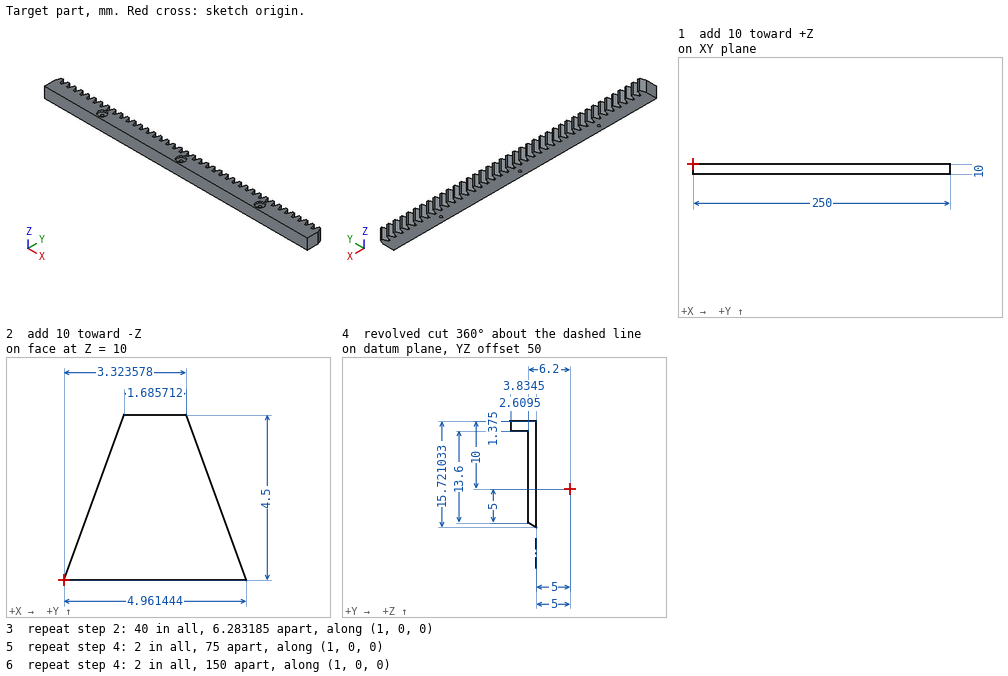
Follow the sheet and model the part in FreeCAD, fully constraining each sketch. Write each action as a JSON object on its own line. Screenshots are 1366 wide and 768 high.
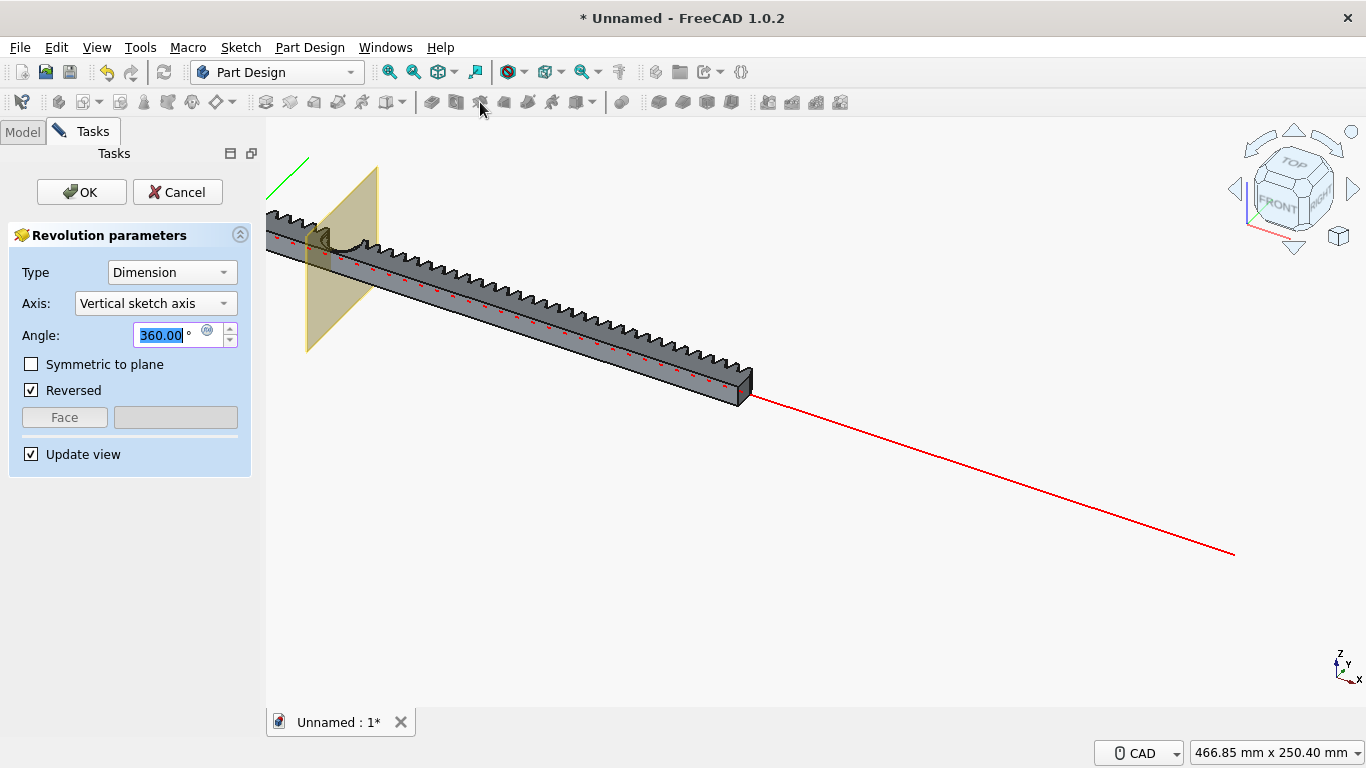
{"action": "left_click", "coordinate": [156, 304]}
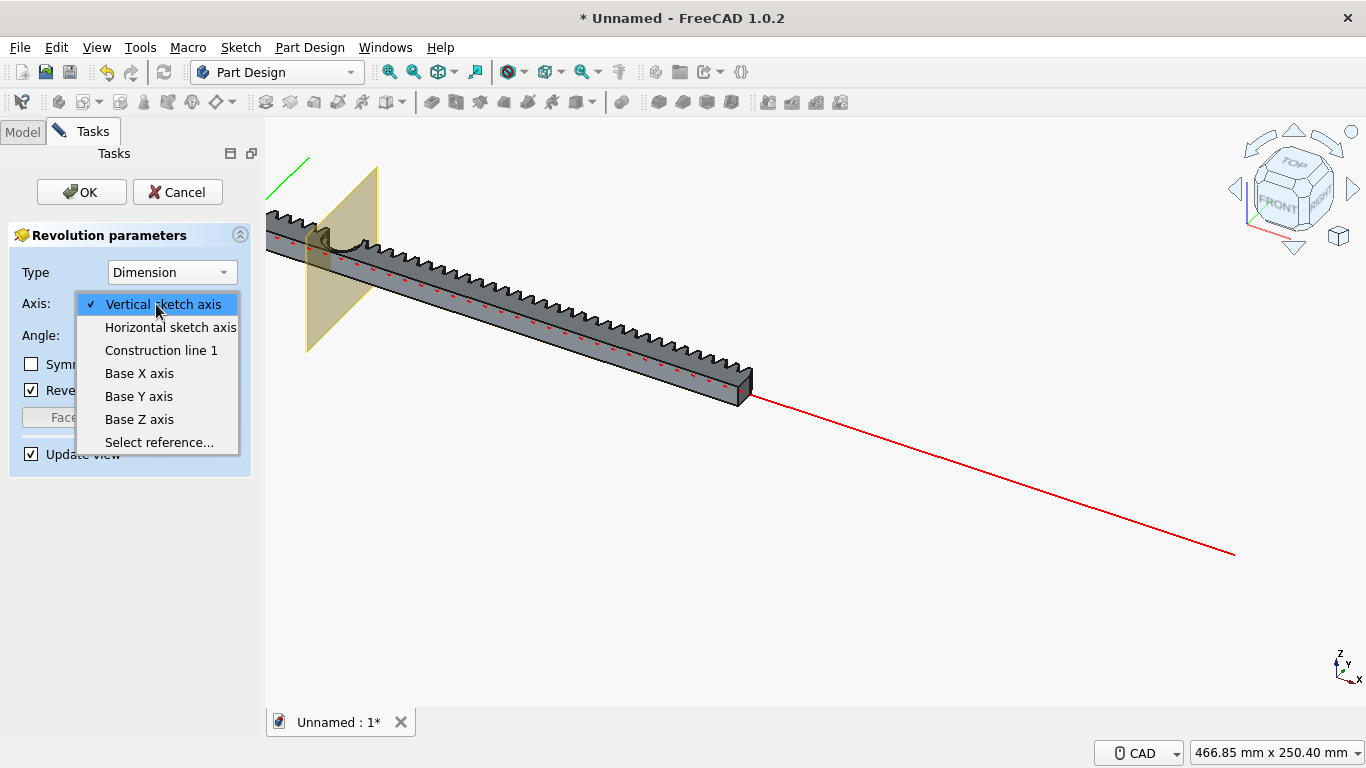
{"action": "left_click", "coordinate": [156, 350]}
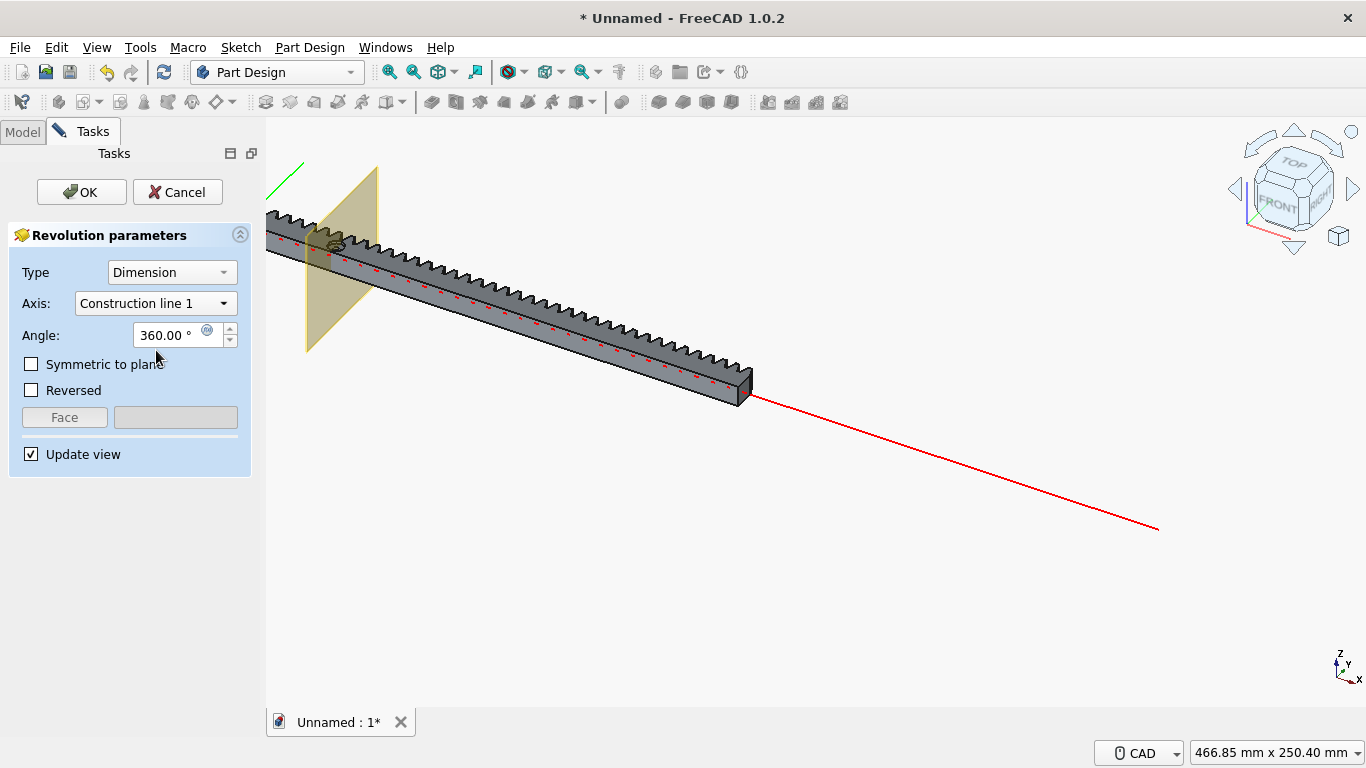
{"action": "left_click", "coordinate": [82, 192]}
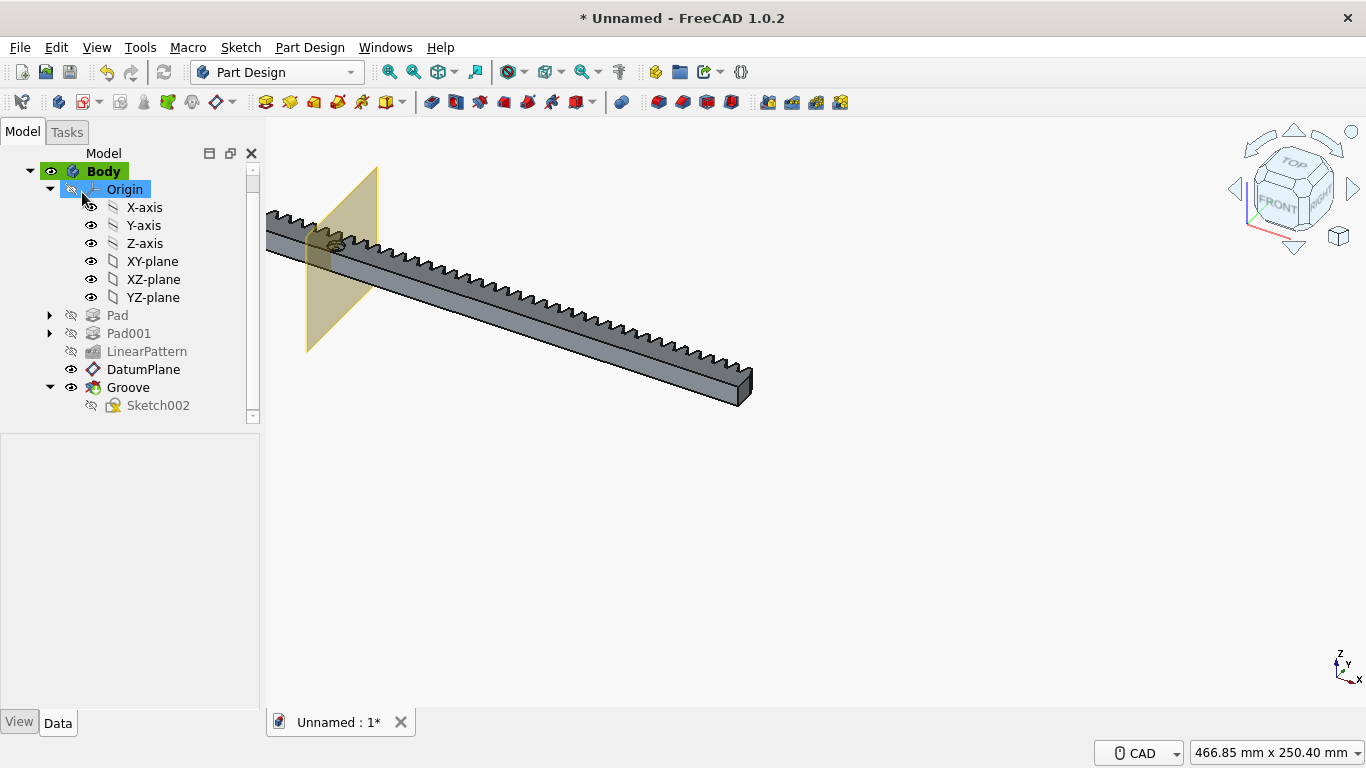
{"action": "left_click", "coordinate": [116, 369]}
{"action": "key", "text": "space"}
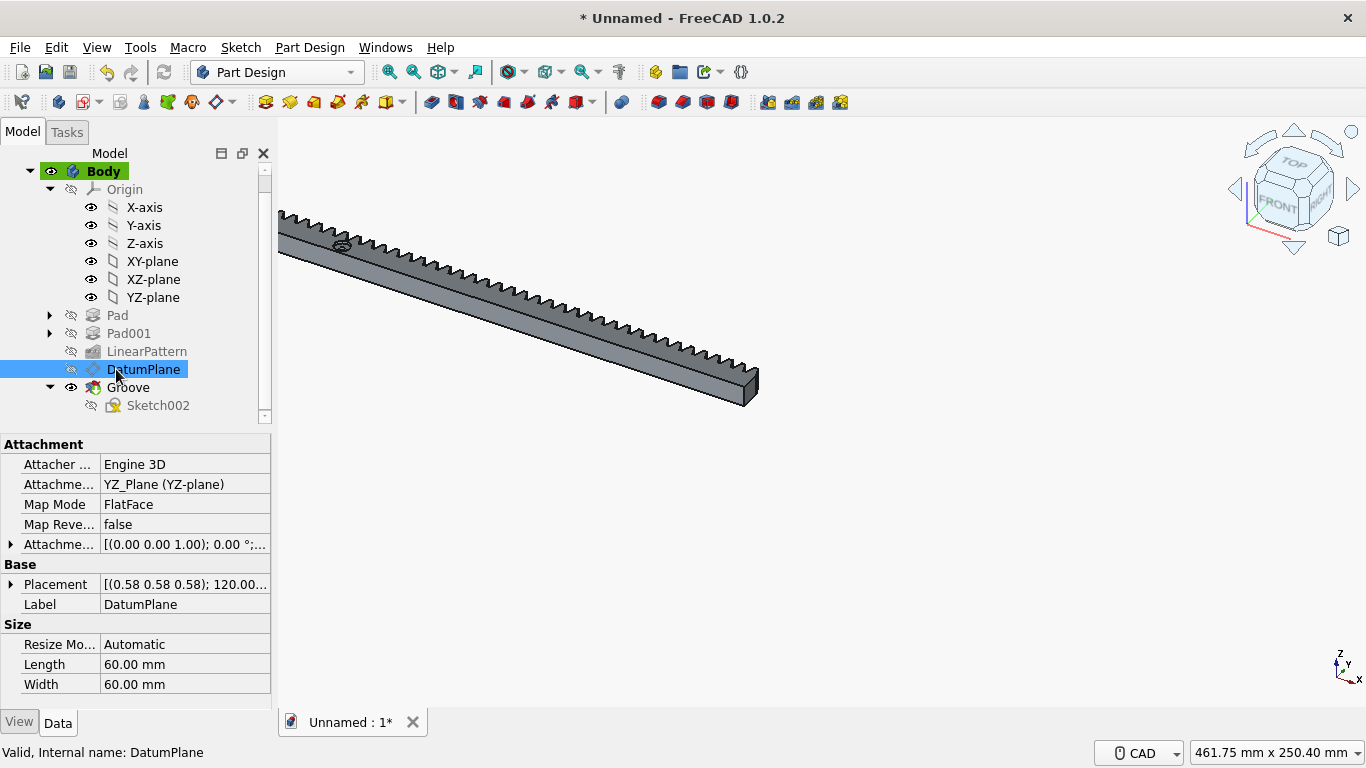
{"action": "left_click", "coordinate": [390, 72]}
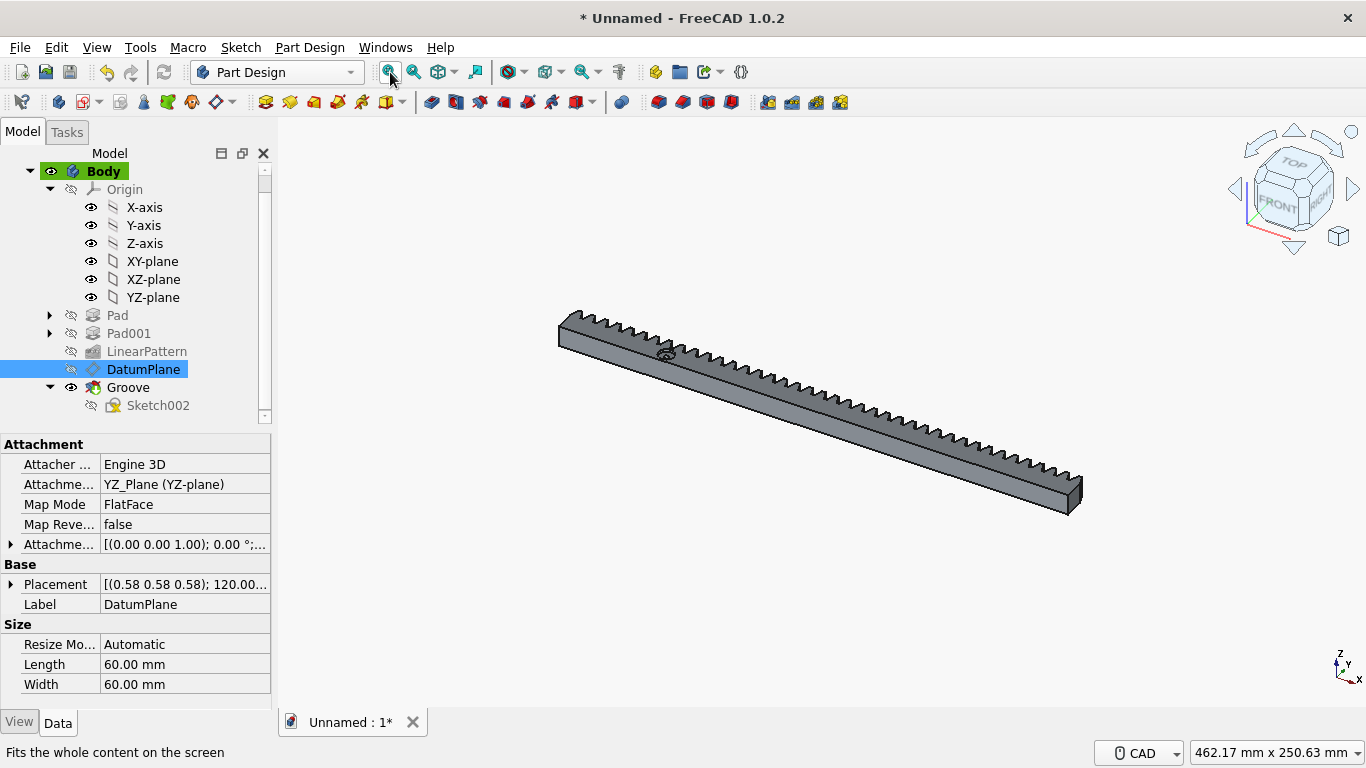
{"action": "left_click", "coordinate": [116, 387]}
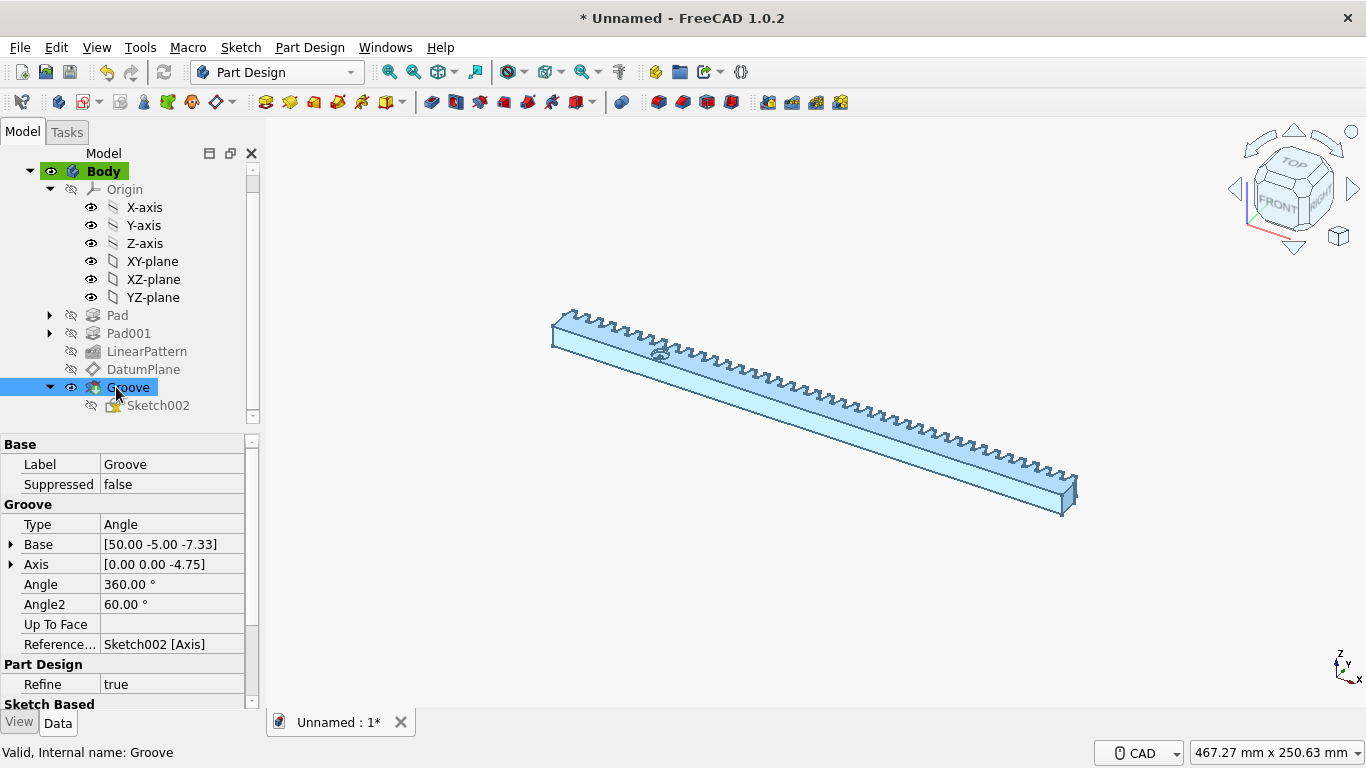
{"action": "left_click", "coordinate": [792, 102]}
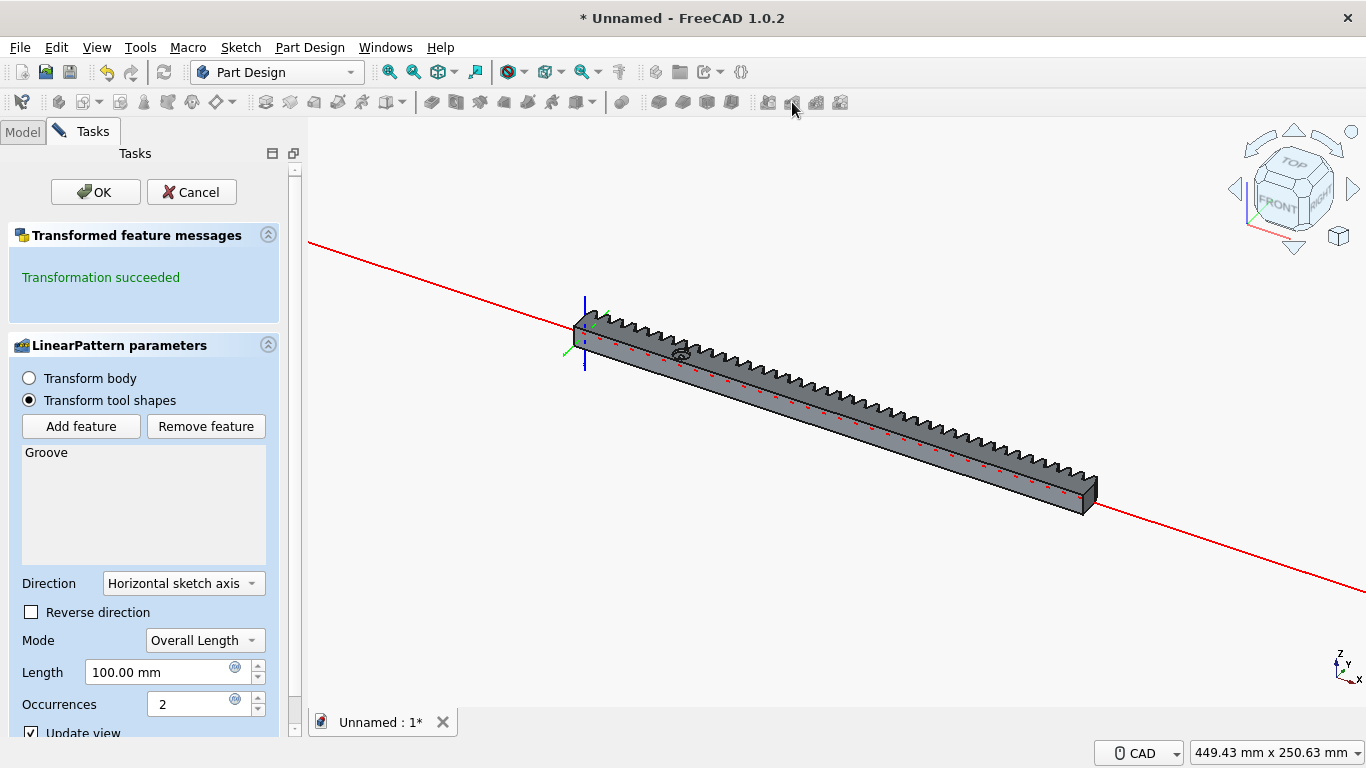
{"action": "left_click", "coordinate": [184, 584]}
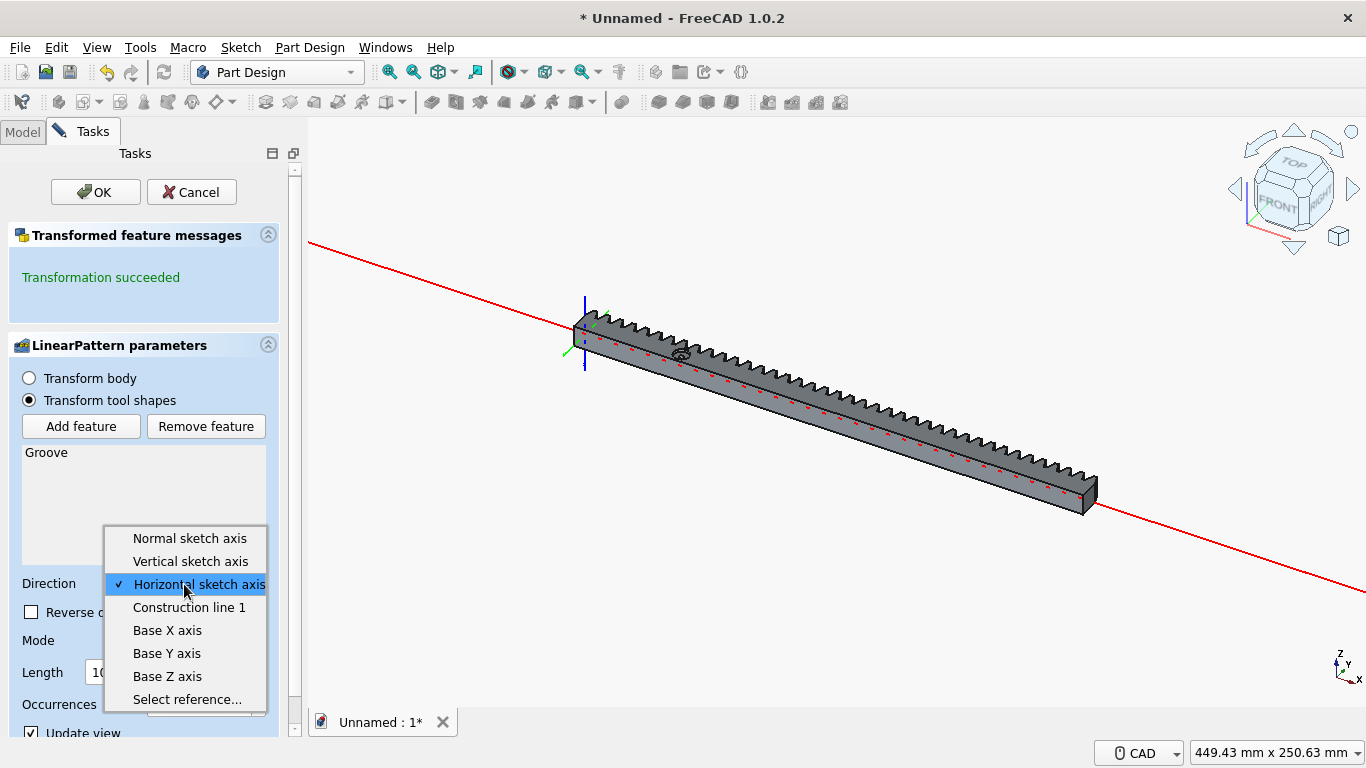
{"action": "left_click", "coordinate": [184, 630]}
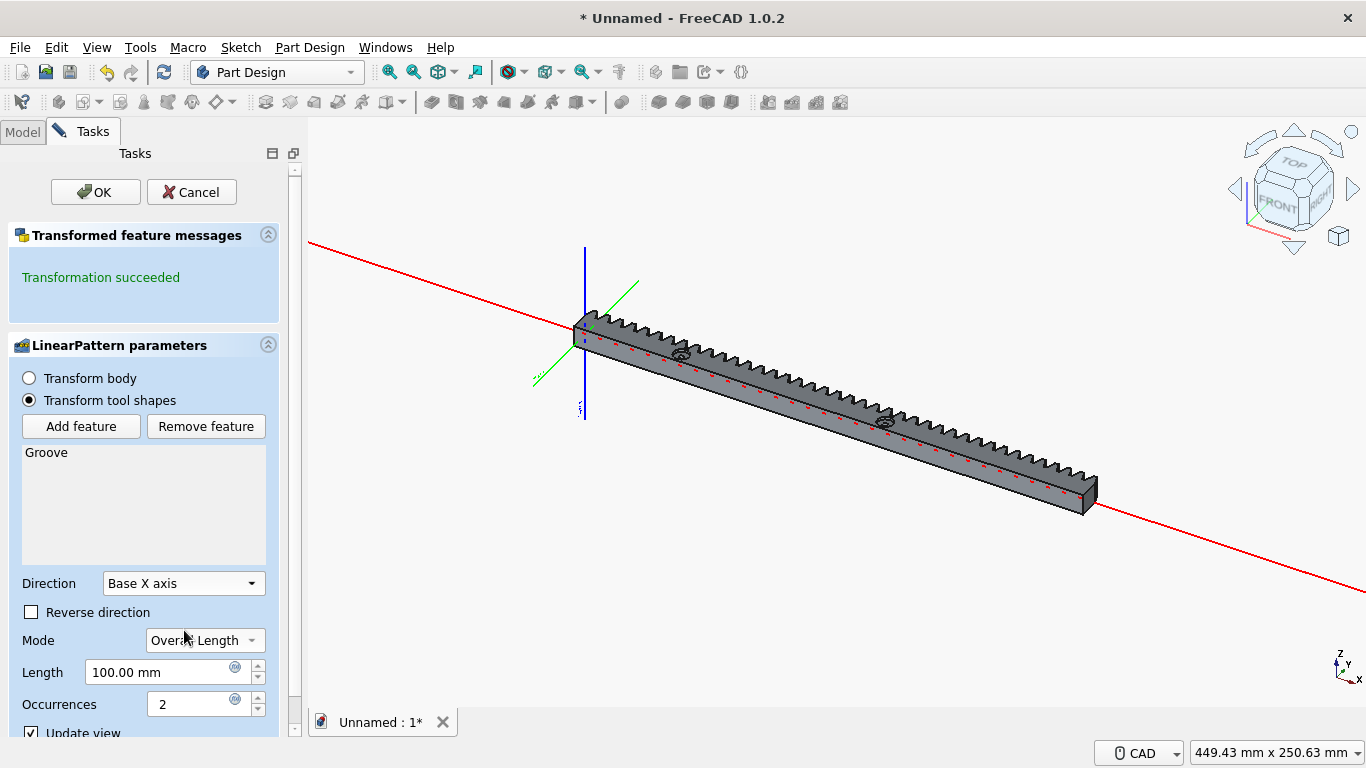
{"action": "left_click", "coordinate": [206, 640]}